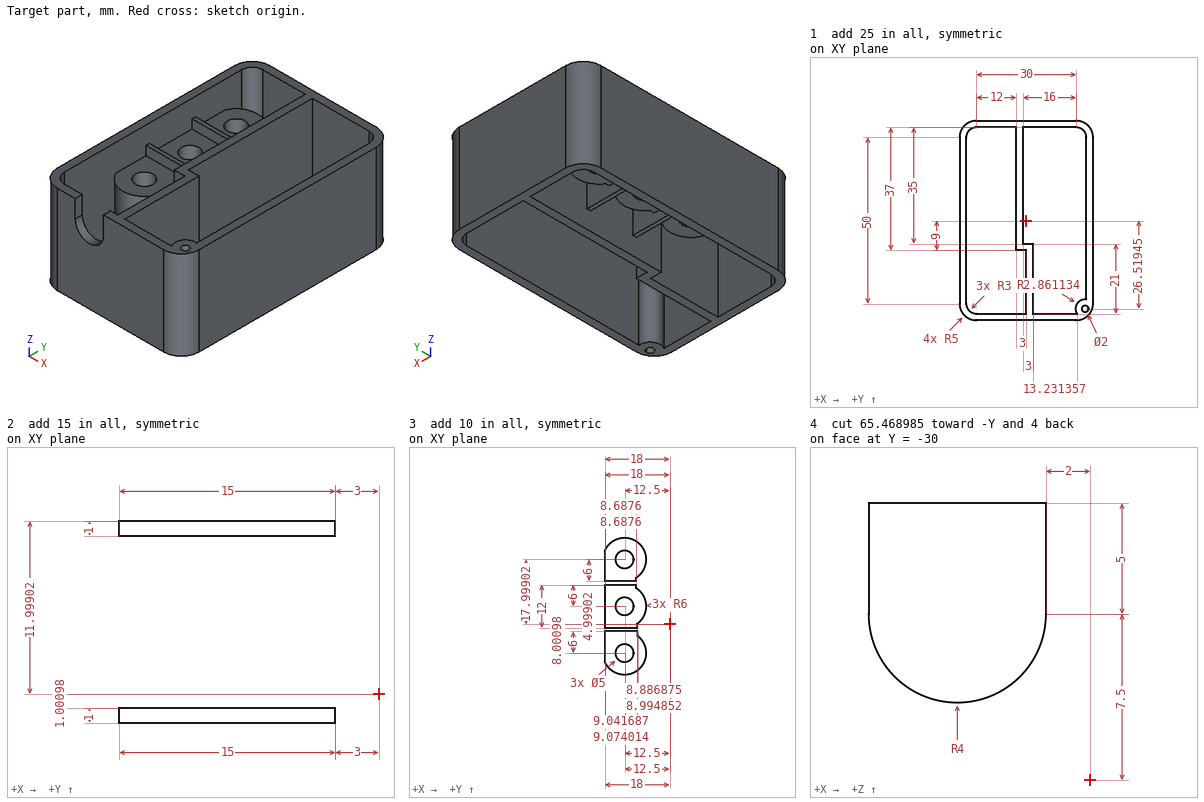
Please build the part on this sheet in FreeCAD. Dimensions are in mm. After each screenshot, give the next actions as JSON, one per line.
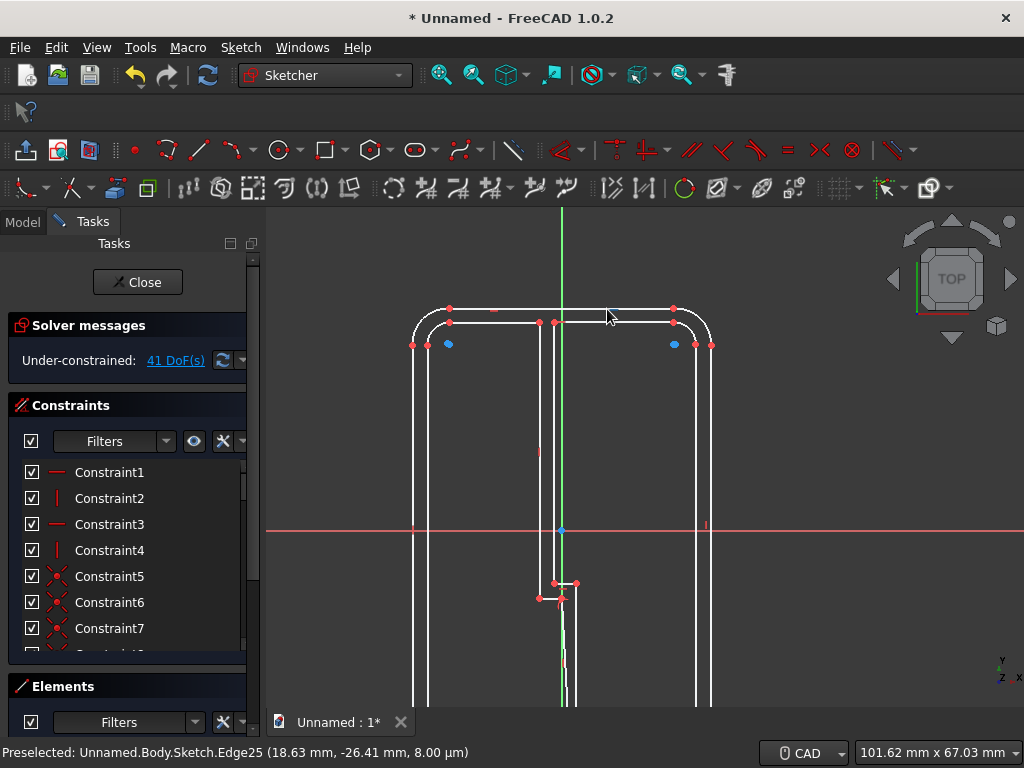
{"action": "left_click", "coordinate": [607, 309]}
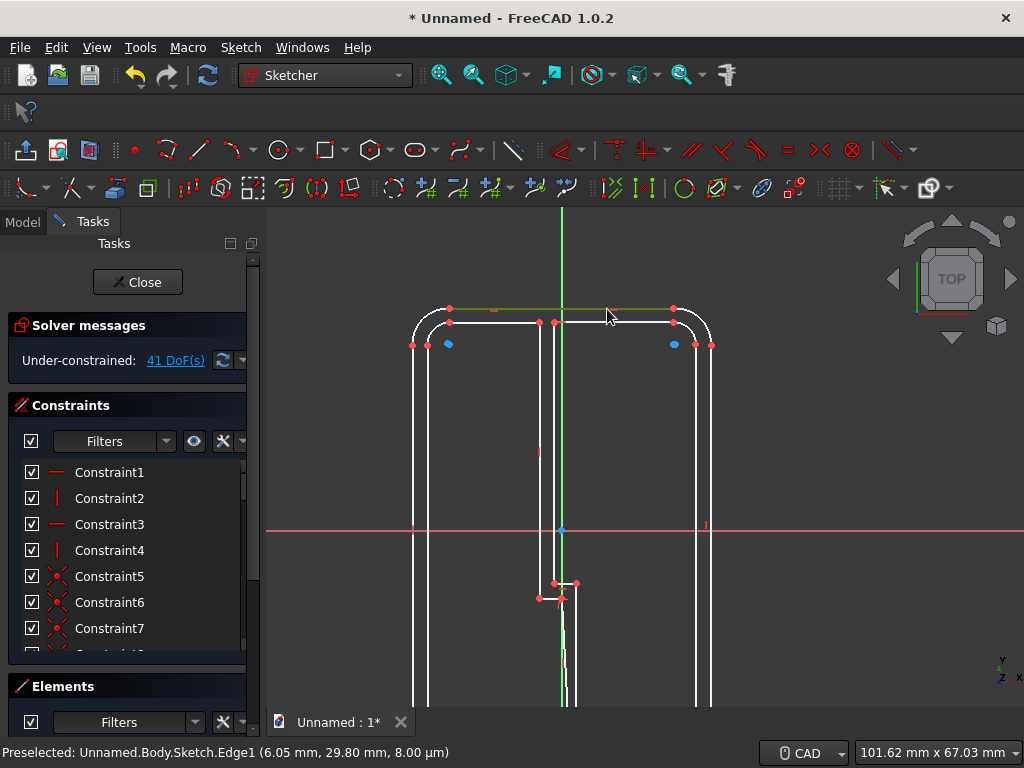
{"action": "left_click", "coordinate": [433, 312]}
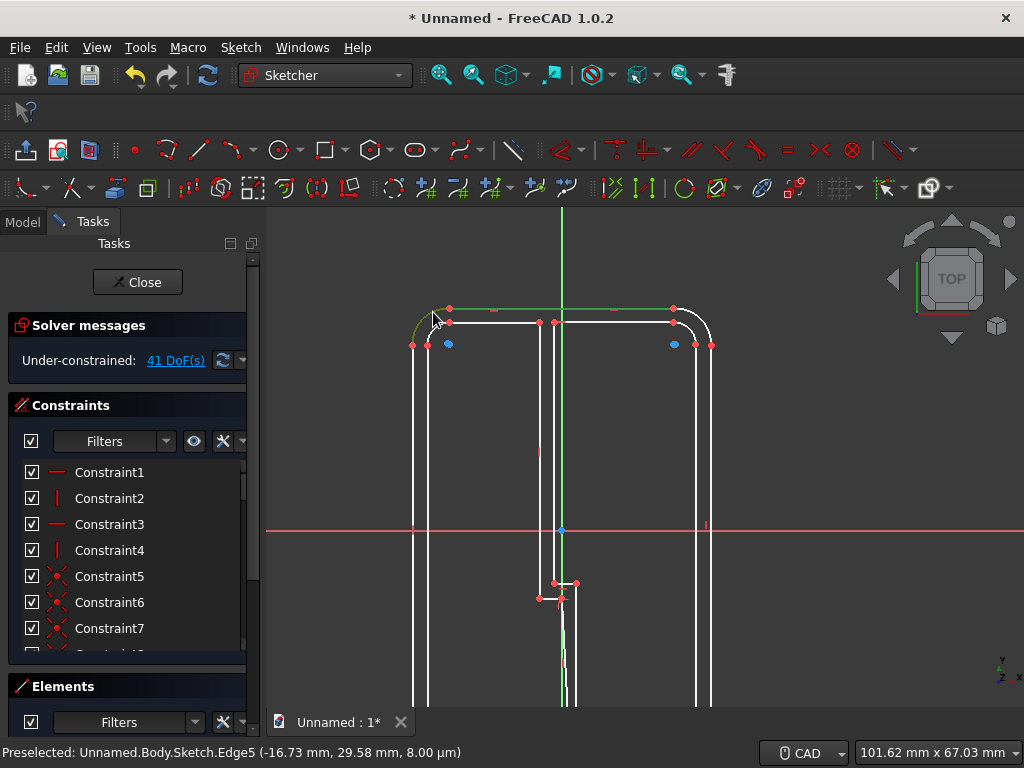
{"action": "left_click", "coordinate": [756, 150]}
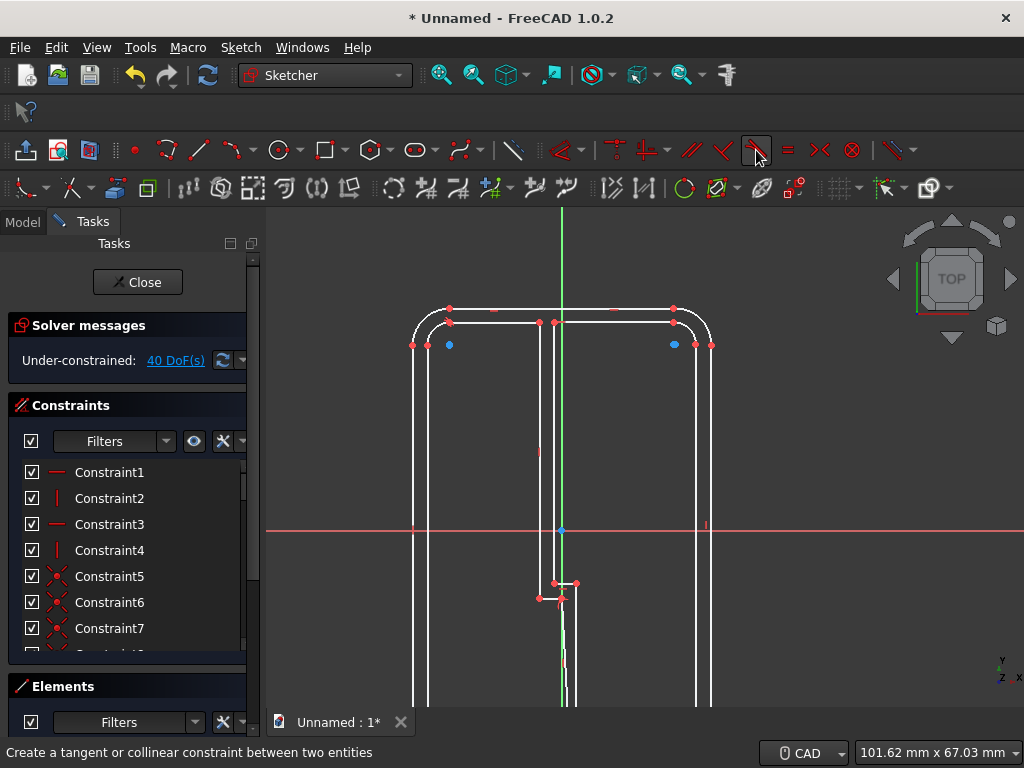
{"action": "left_click", "coordinate": [607, 309]}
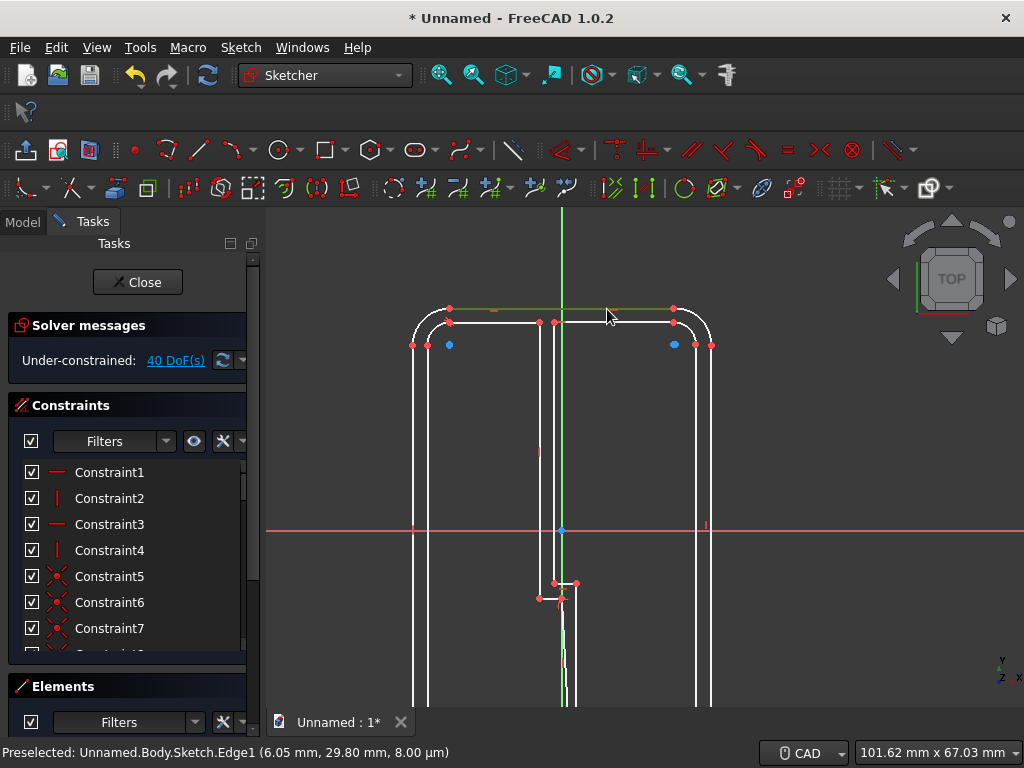
{"action": "left_click", "coordinate": [708, 329]}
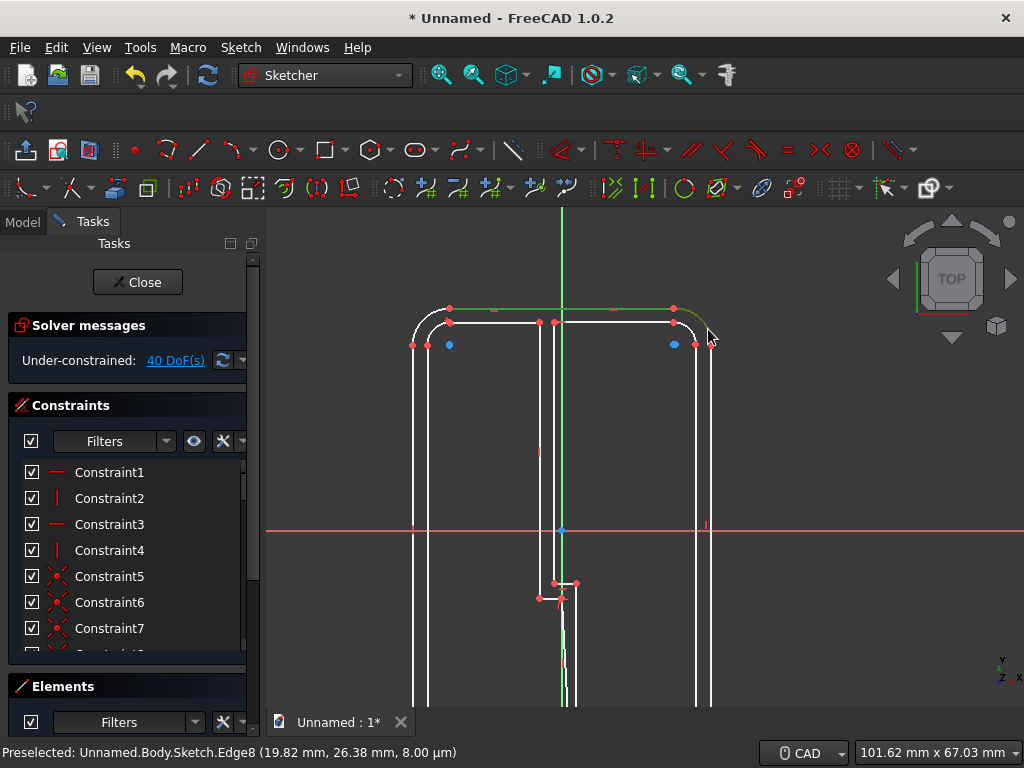
{"action": "left_click", "coordinate": [756, 150]}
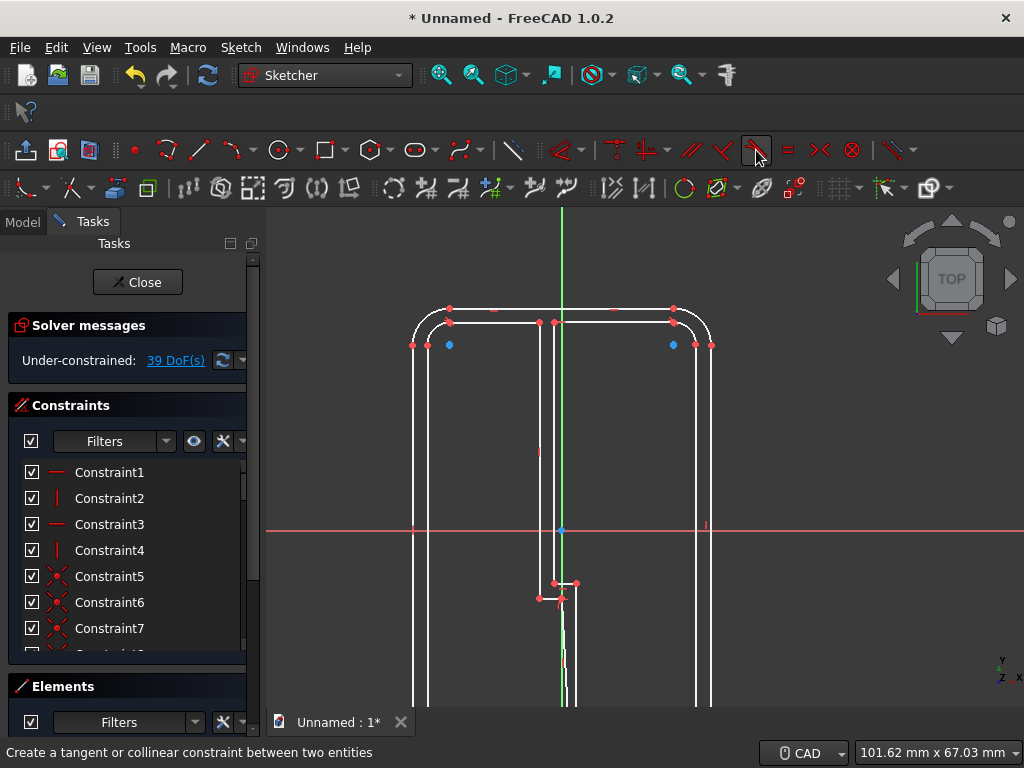
{"action": "left_click", "coordinate": [413, 458]}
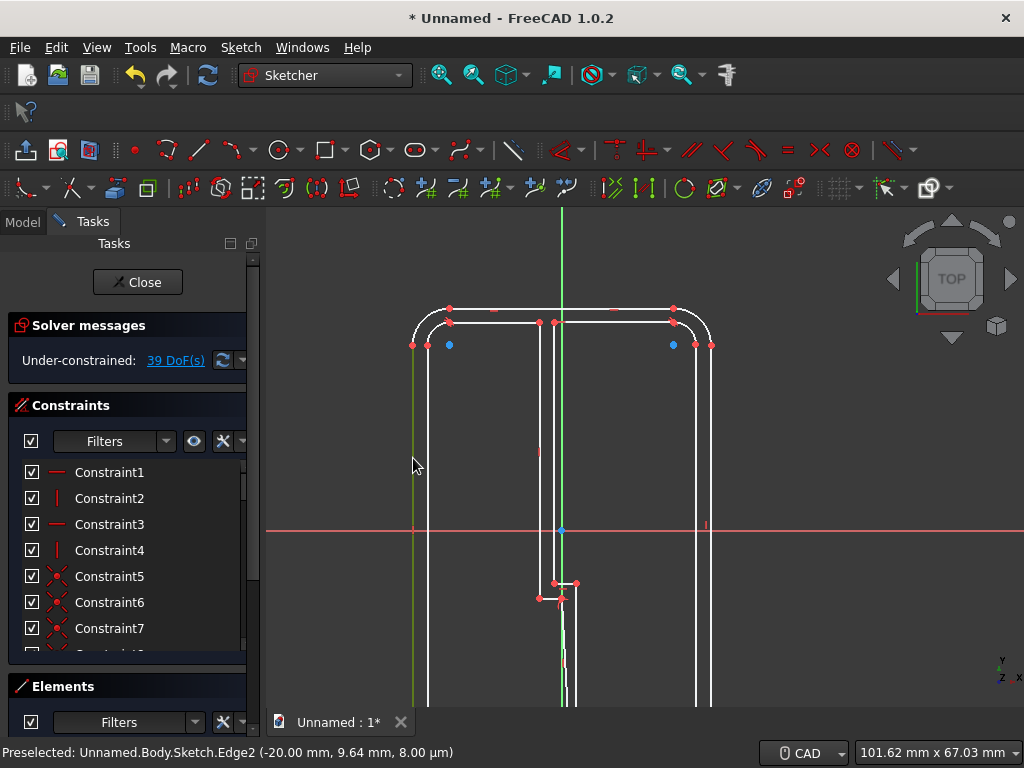
{"action": "left_click", "coordinate": [433, 313]}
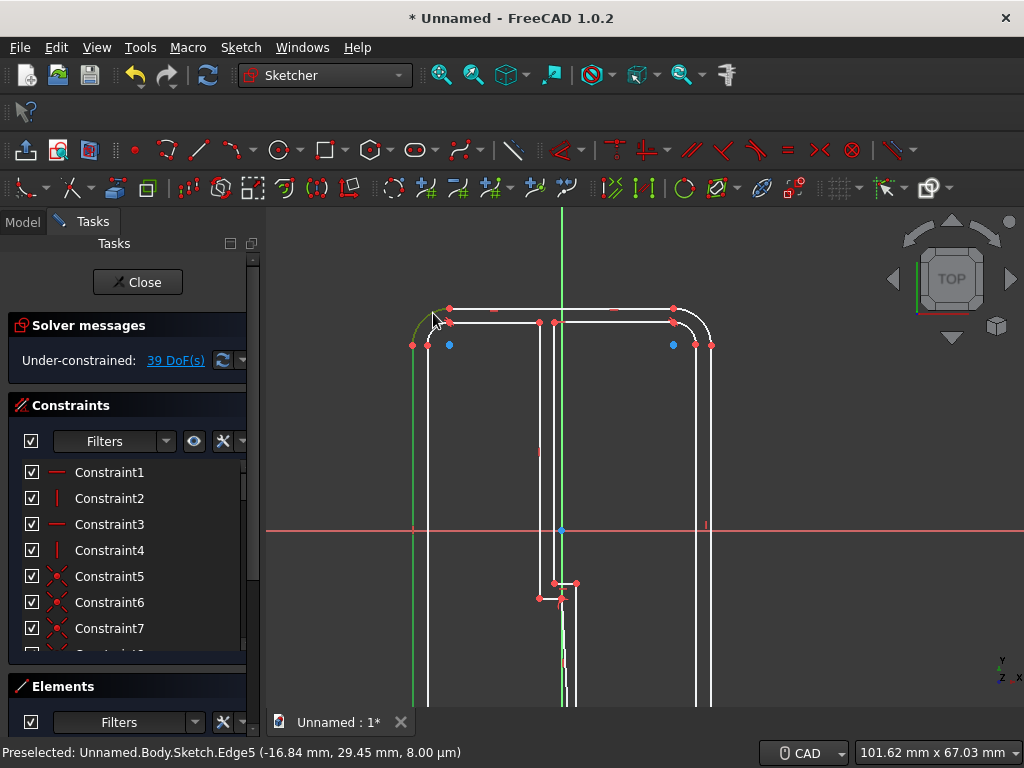
{"action": "left_click", "coordinate": [756, 150]}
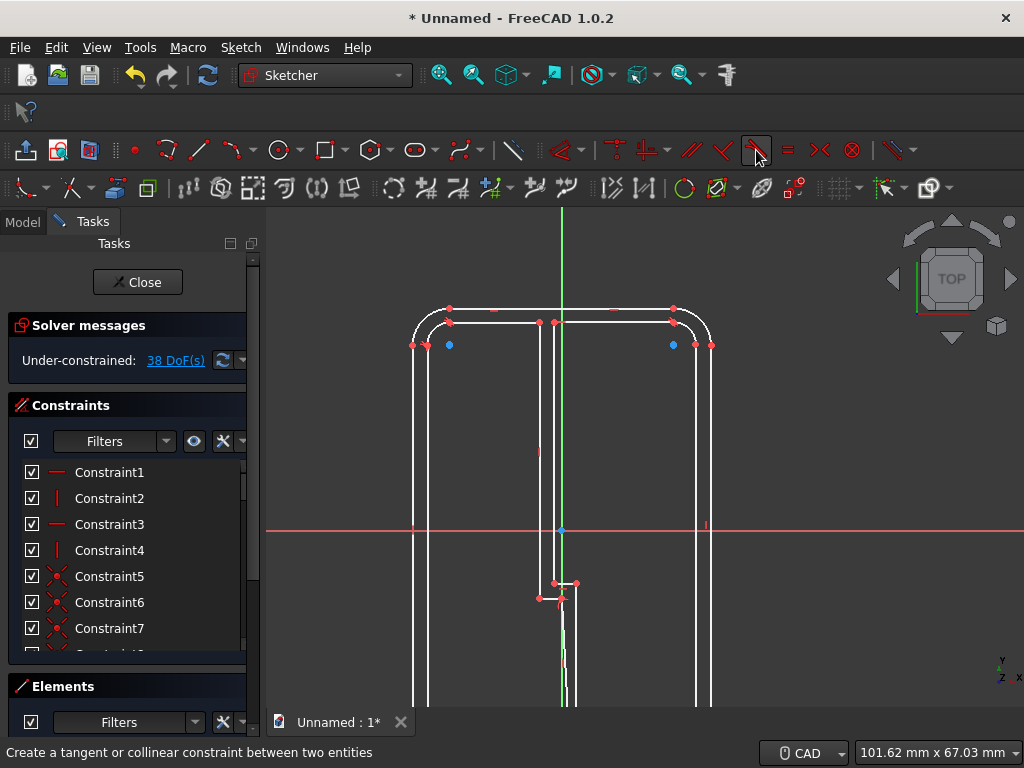
{"action": "left_click", "coordinate": [413, 458]}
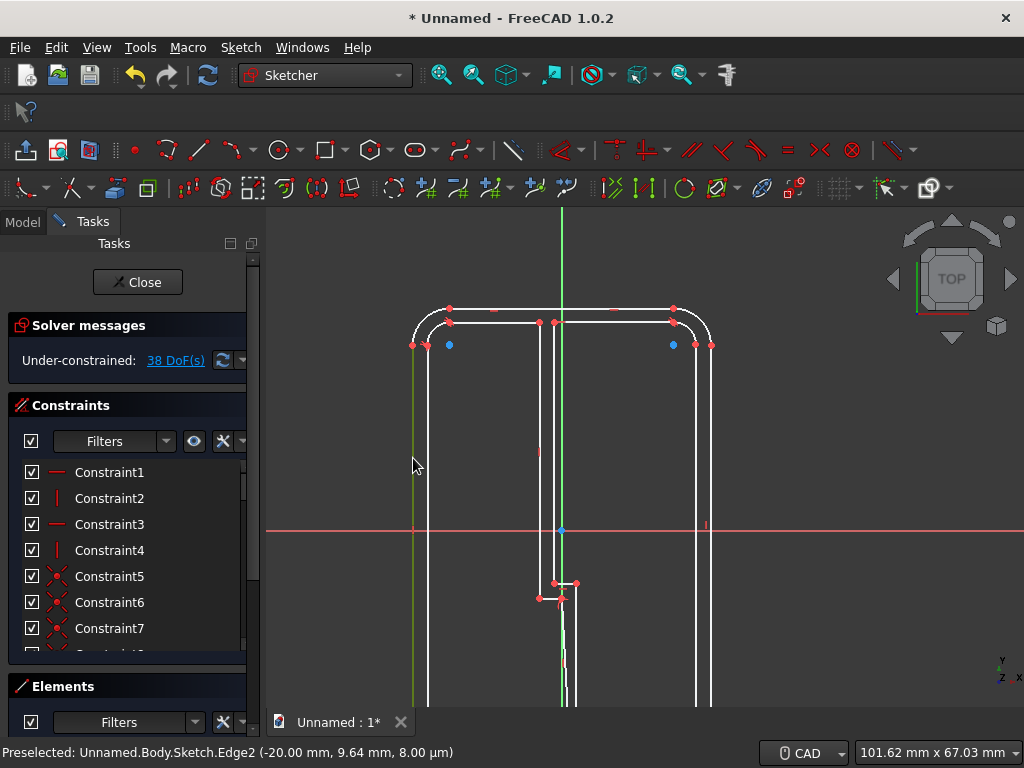
{"action": "scroll", "coordinate": [606, 307], "scroll_direction": "down", "scroll_amount": 2}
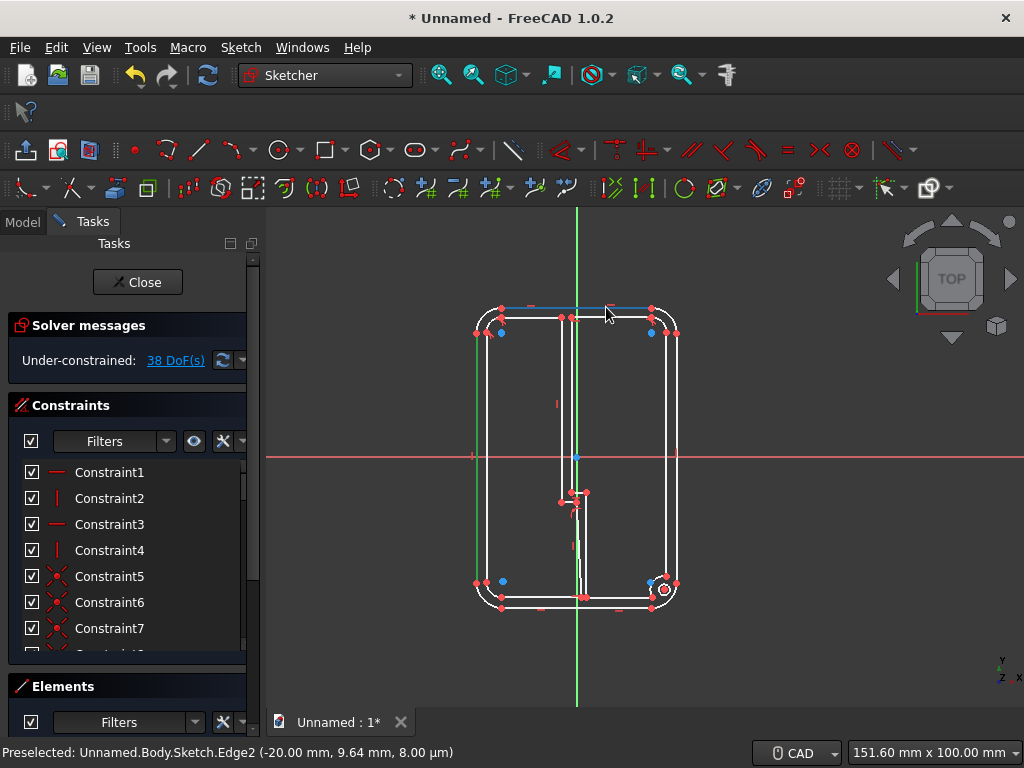
{"action": "scroll", "coordinate": [480, 594], "scroll_direction": "up", "scroll_amount": 2}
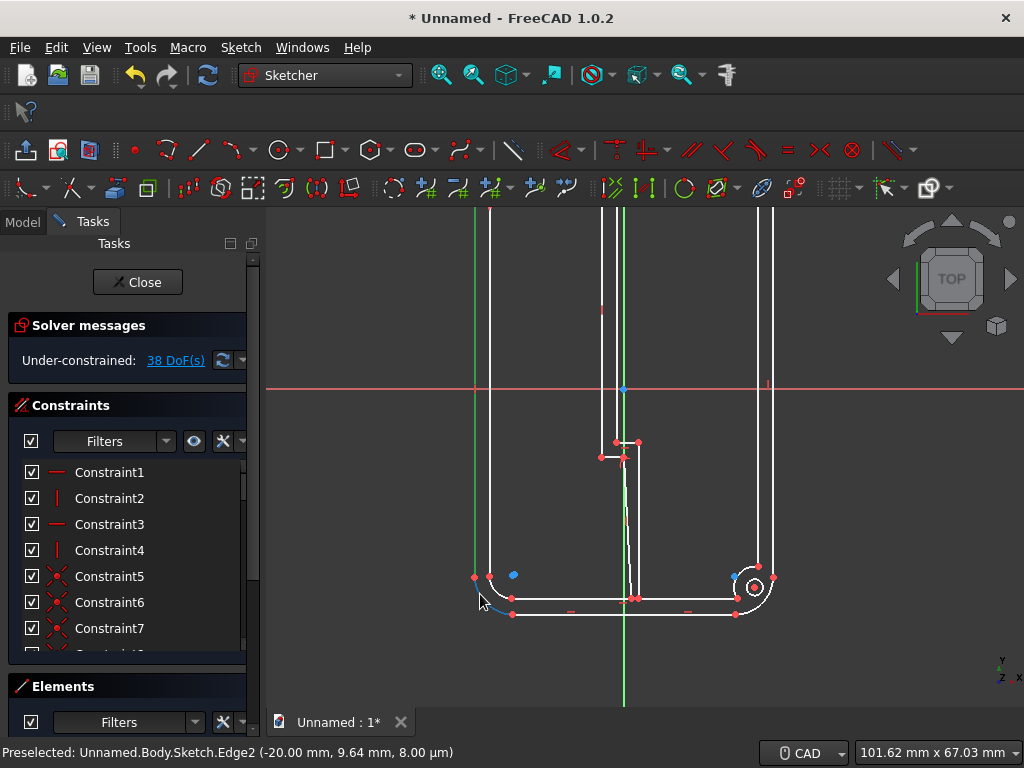
{"action": "left_click", "coordinate": [479, 594]}